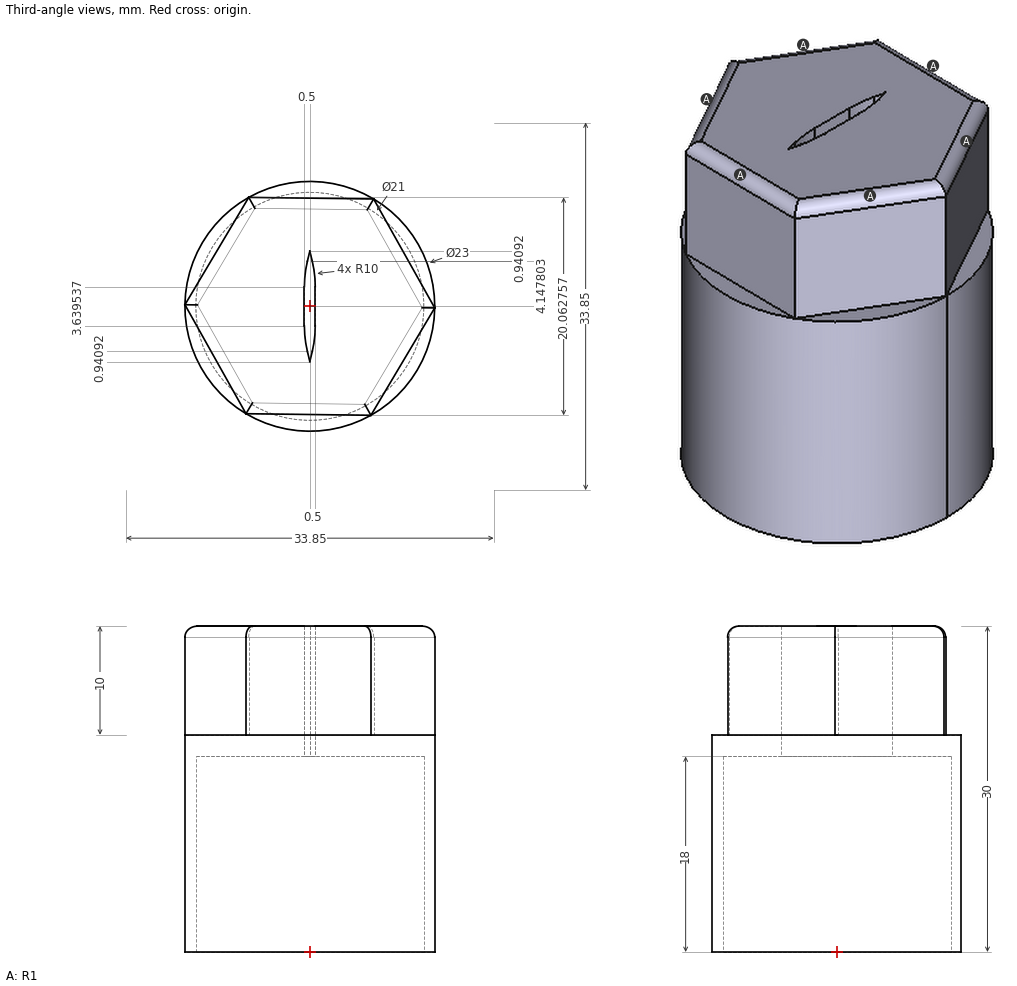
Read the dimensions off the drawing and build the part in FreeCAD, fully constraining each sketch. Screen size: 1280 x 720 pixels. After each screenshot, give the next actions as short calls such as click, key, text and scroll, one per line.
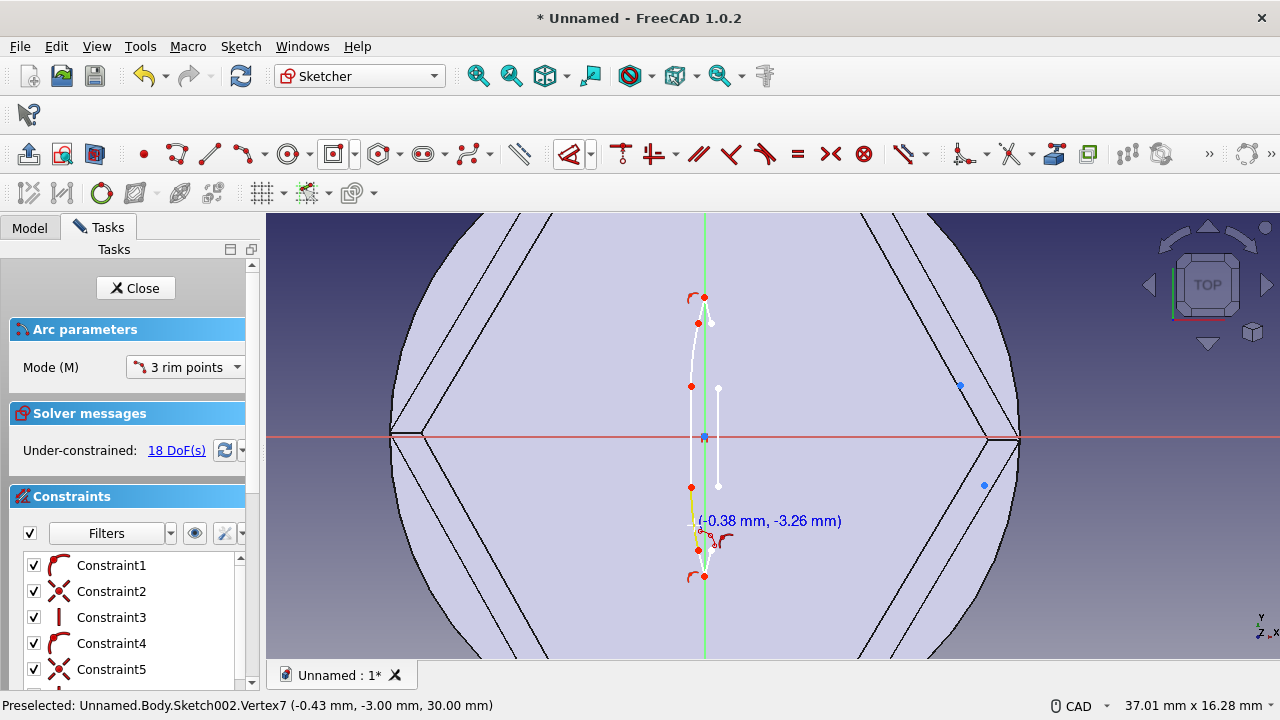
scroll(711, 550, up, 5)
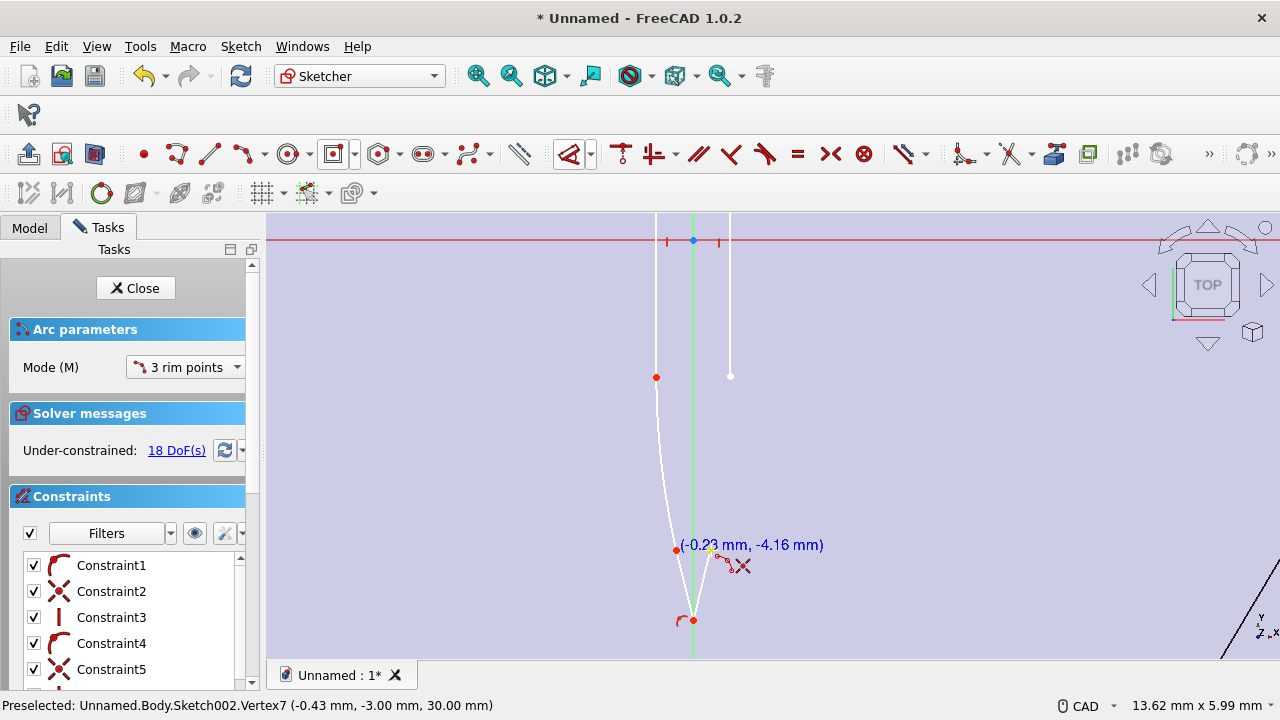
click(710, 550)
click(730, 376)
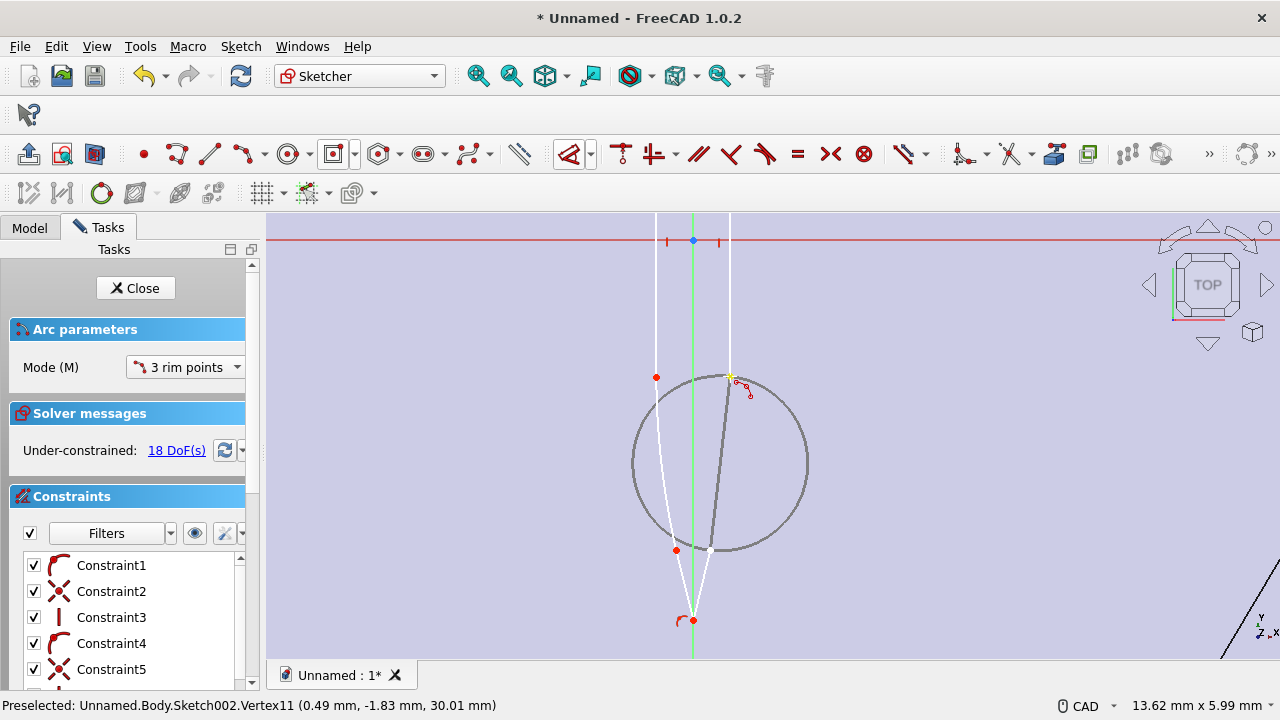
scroll(726, 463, up, 6)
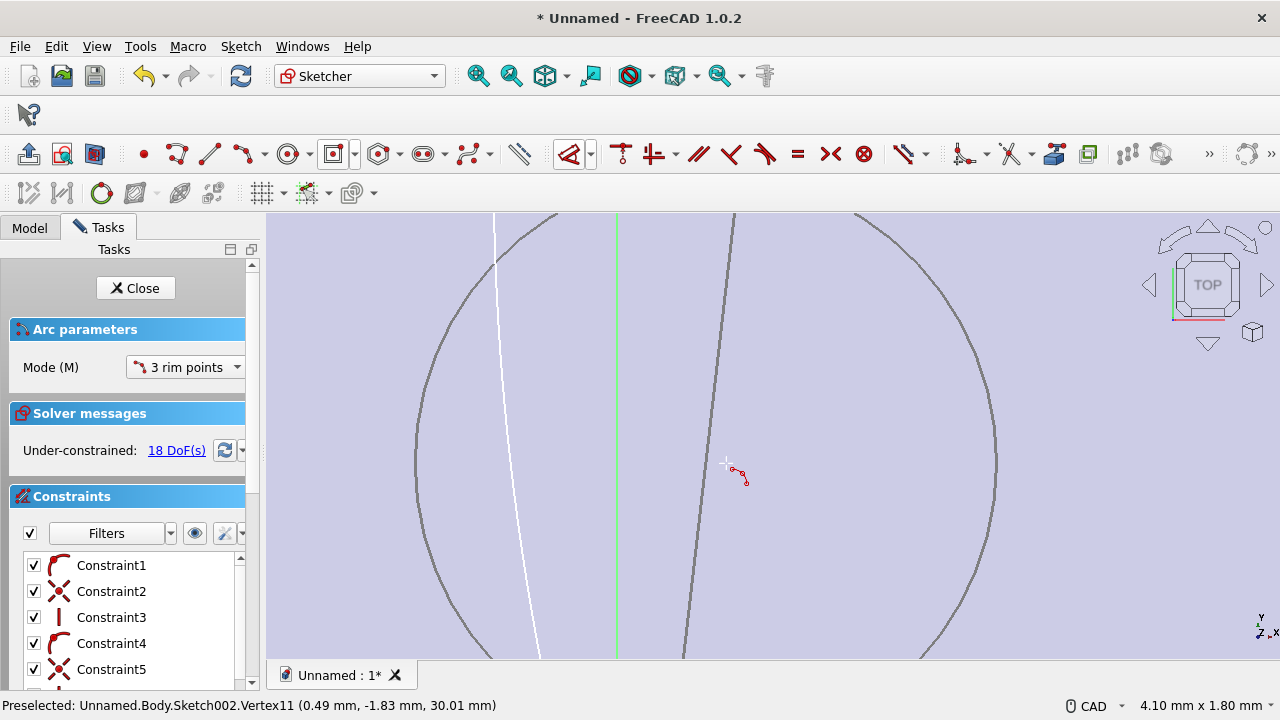
click(724, 462)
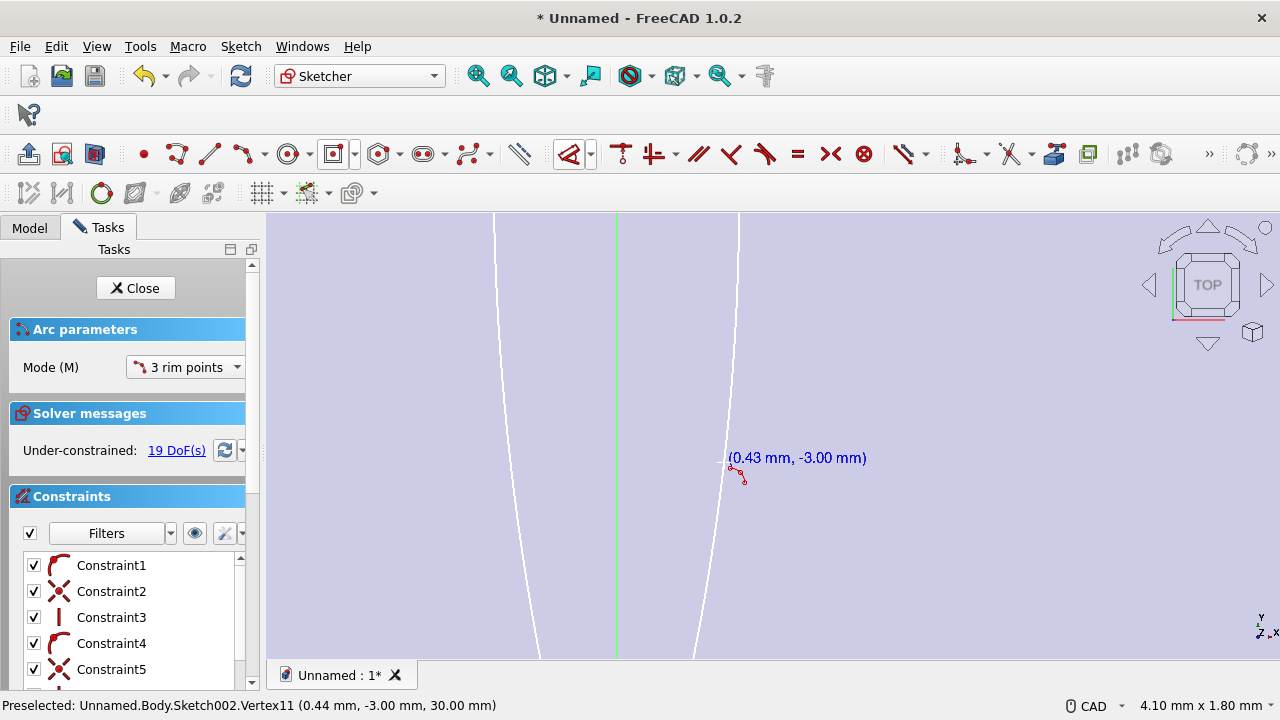
scroll(715, 525, down, 11)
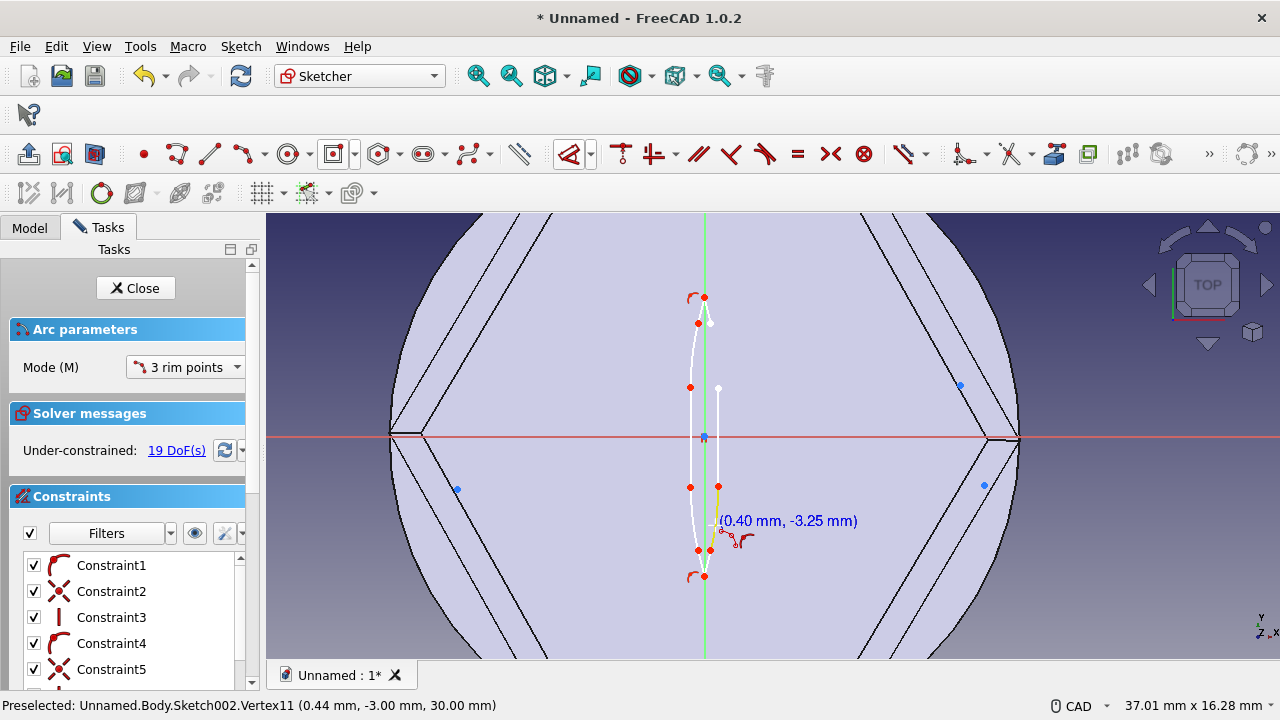
click(718, 388)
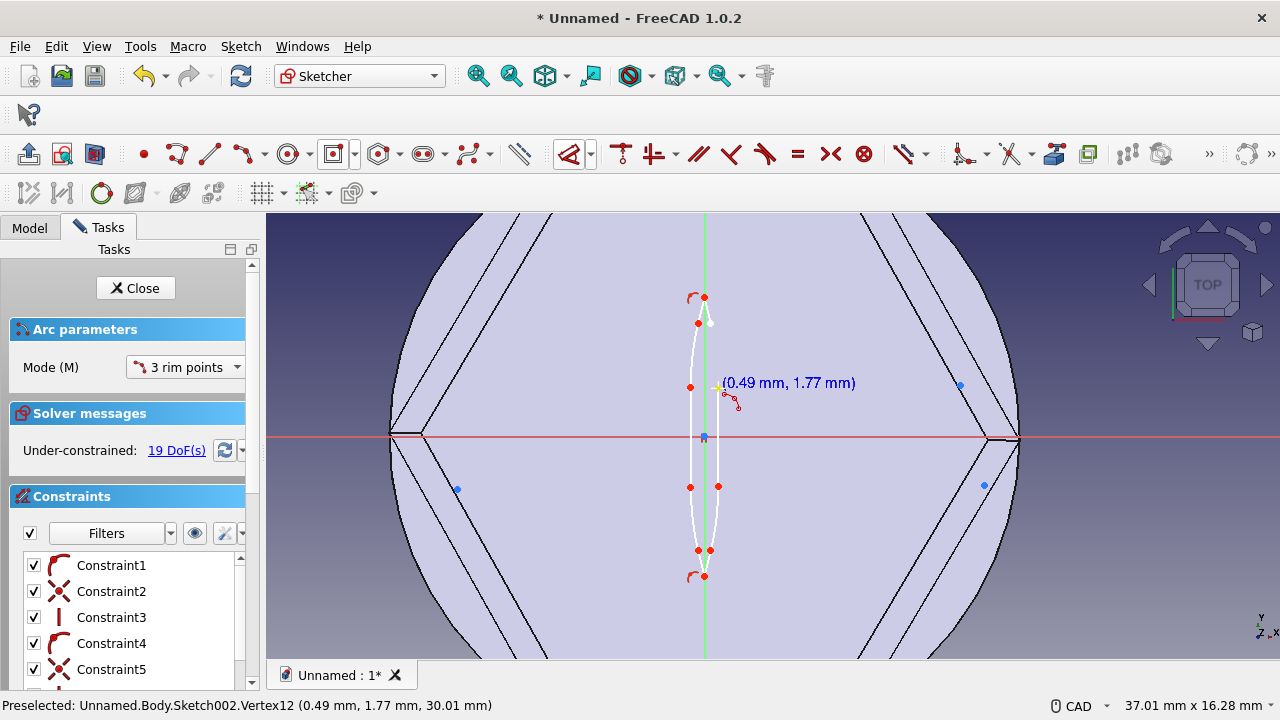
scroll(711, 323, up, 5)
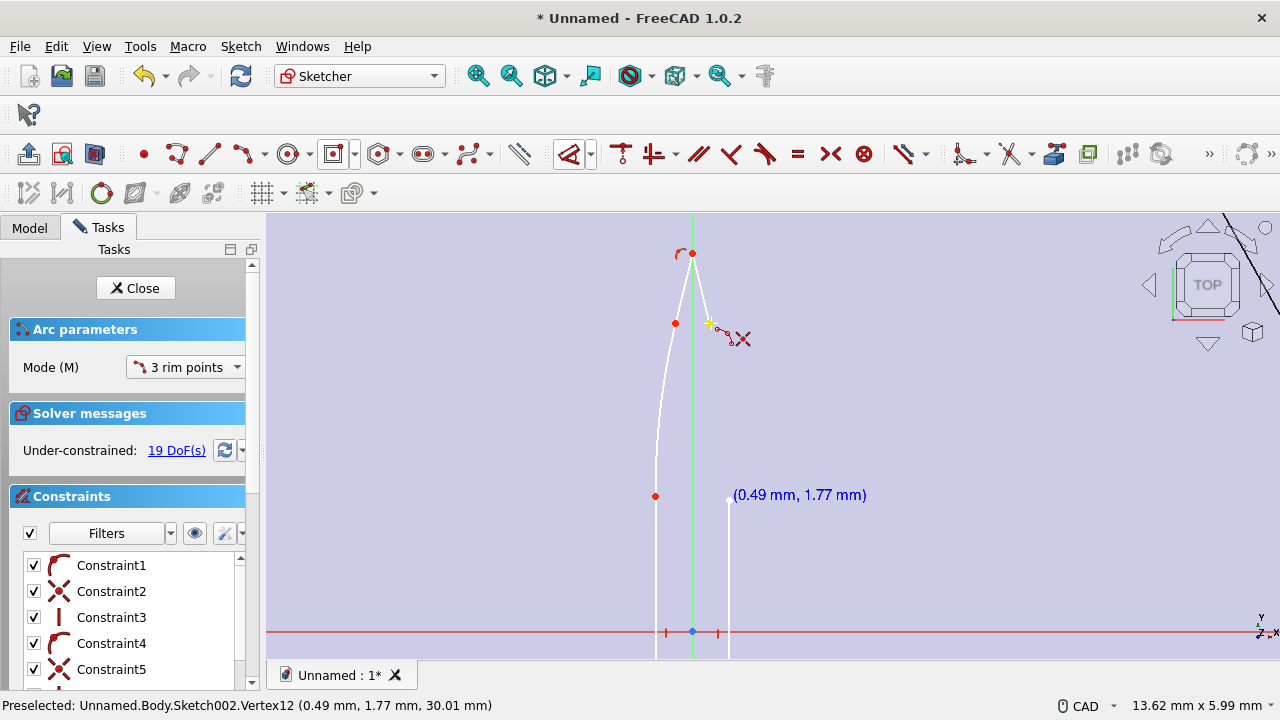
click(710, 324)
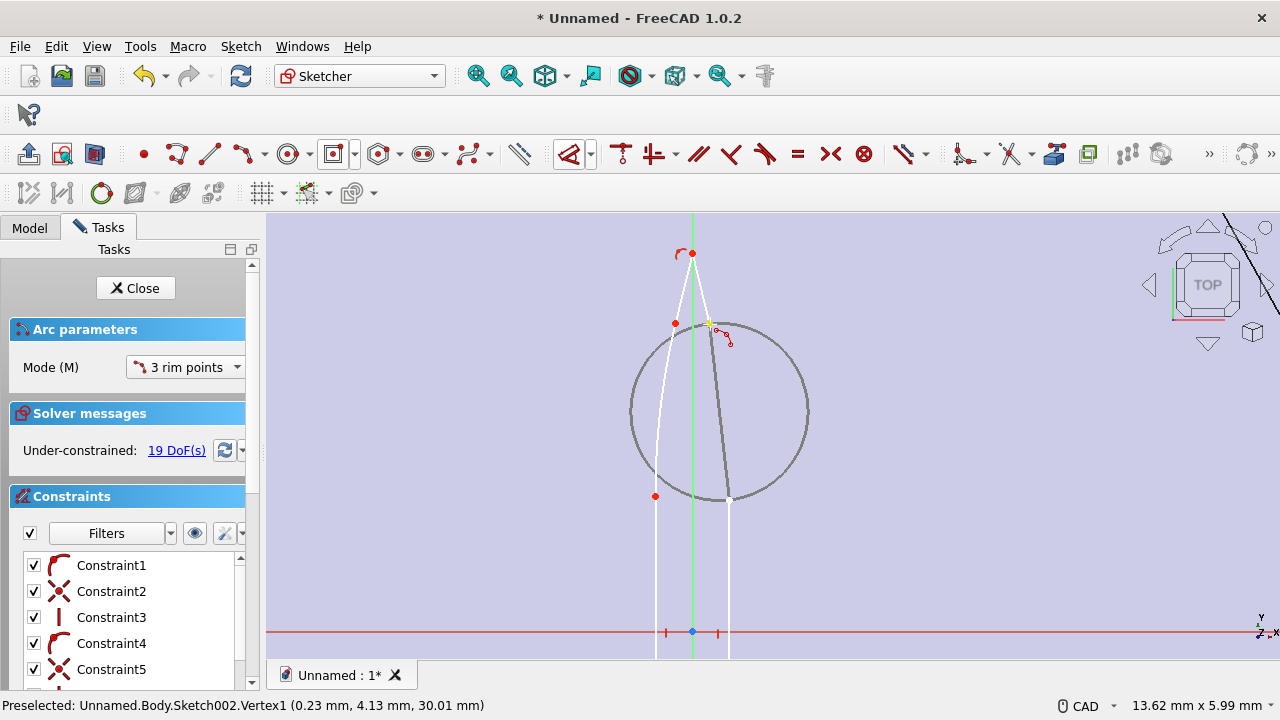
scroll(725, 409, up, 6)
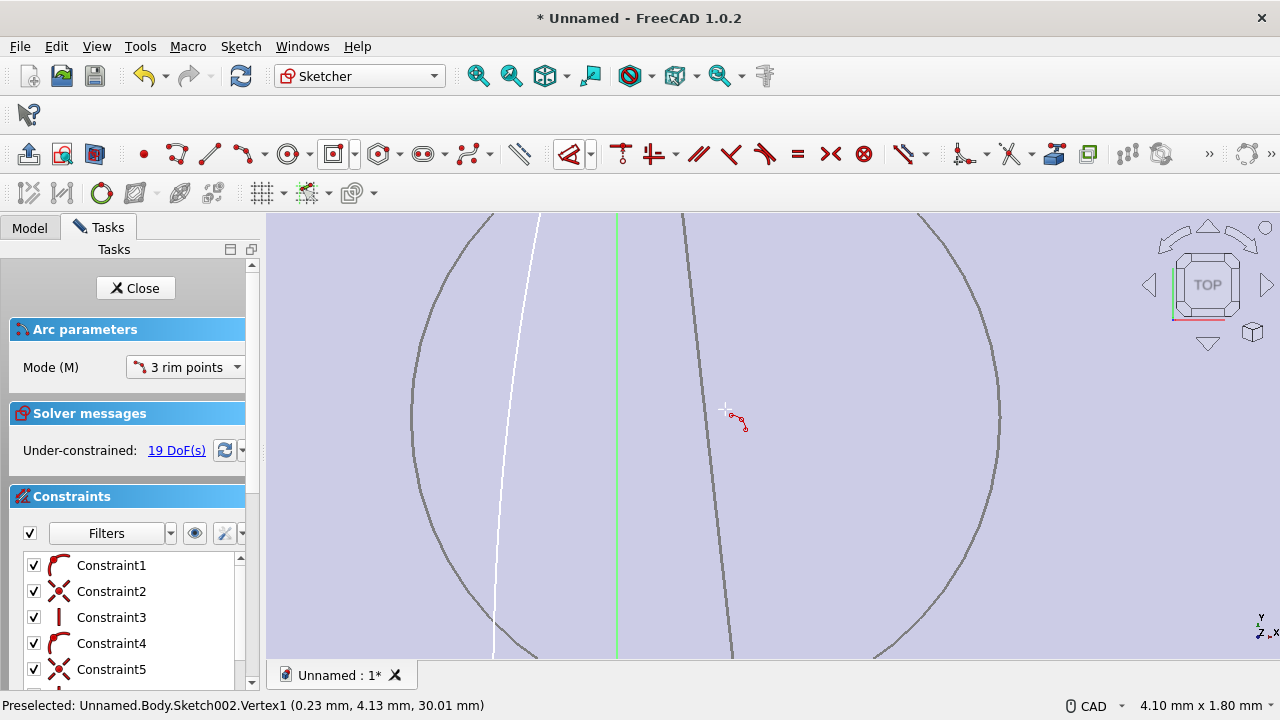
click(723, 407)
key(Escape)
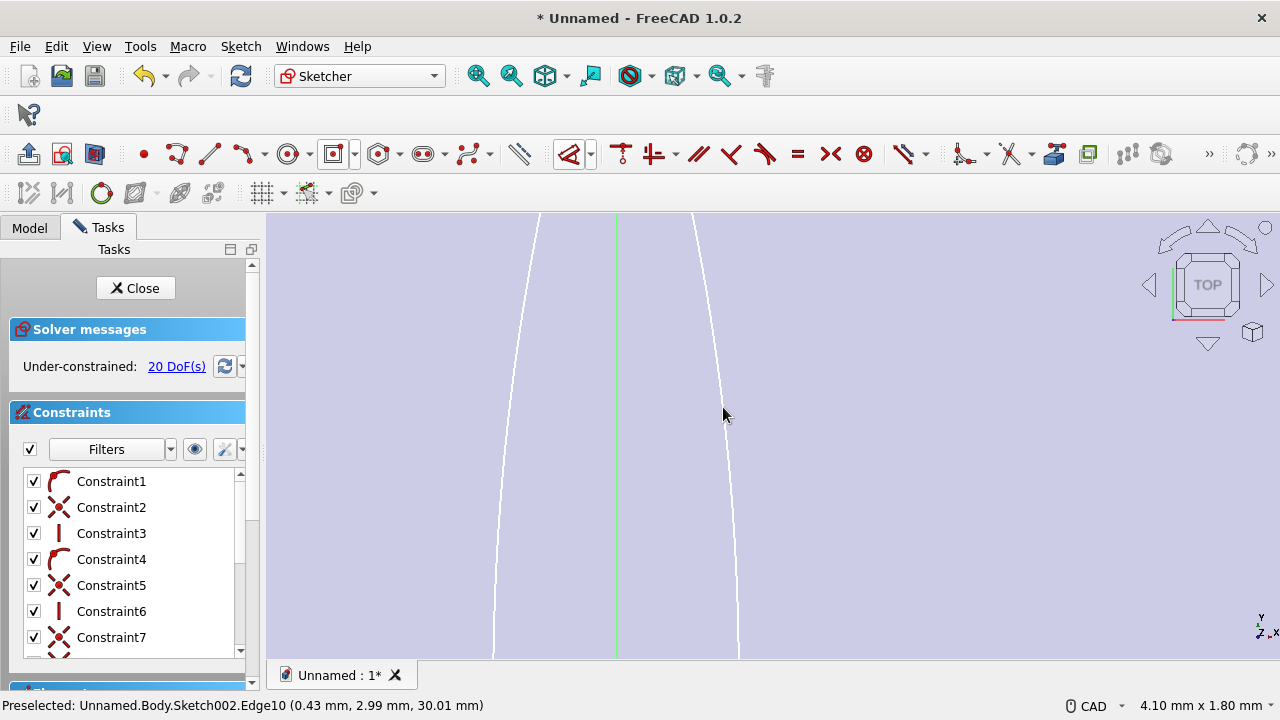
scroll(715, 347, down, 11)